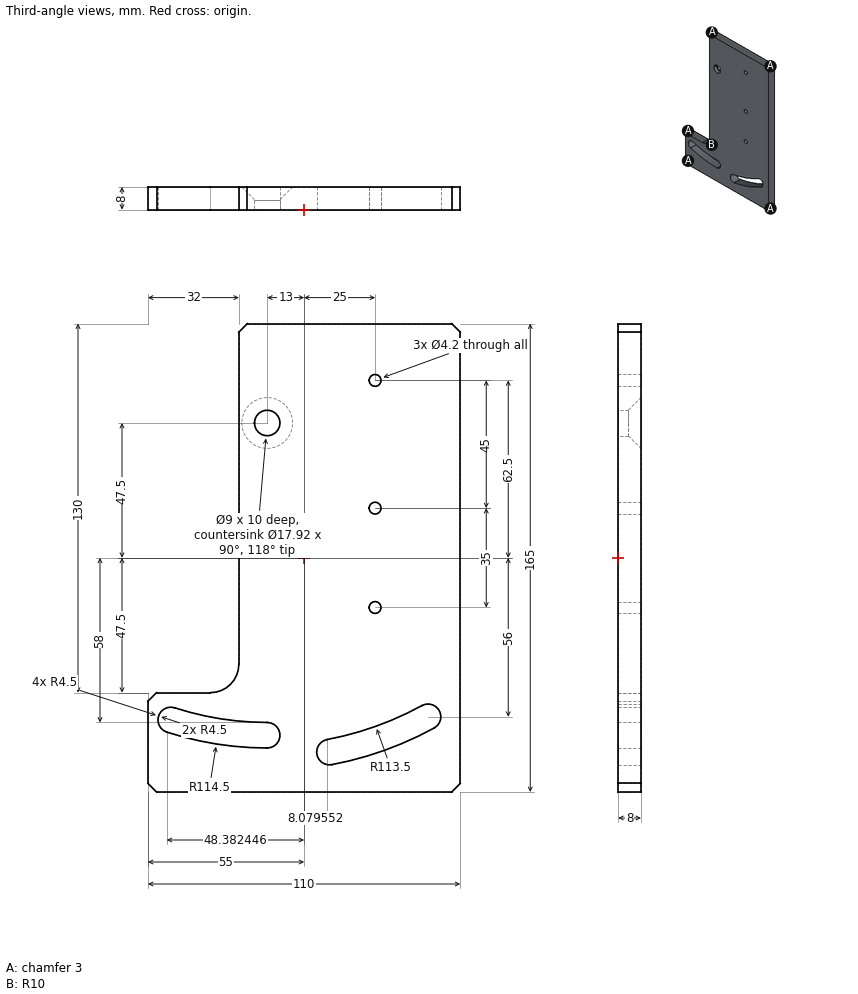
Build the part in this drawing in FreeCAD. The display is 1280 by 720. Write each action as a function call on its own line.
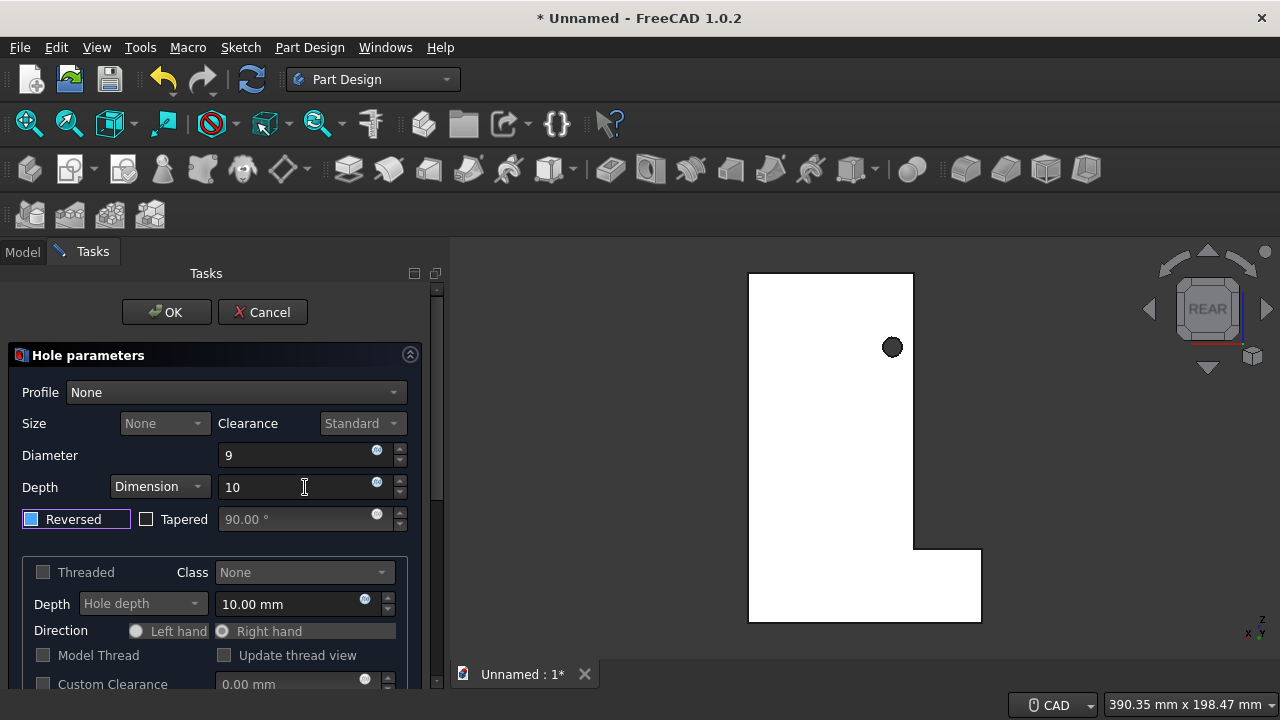
scroll(437, 486, down, 3)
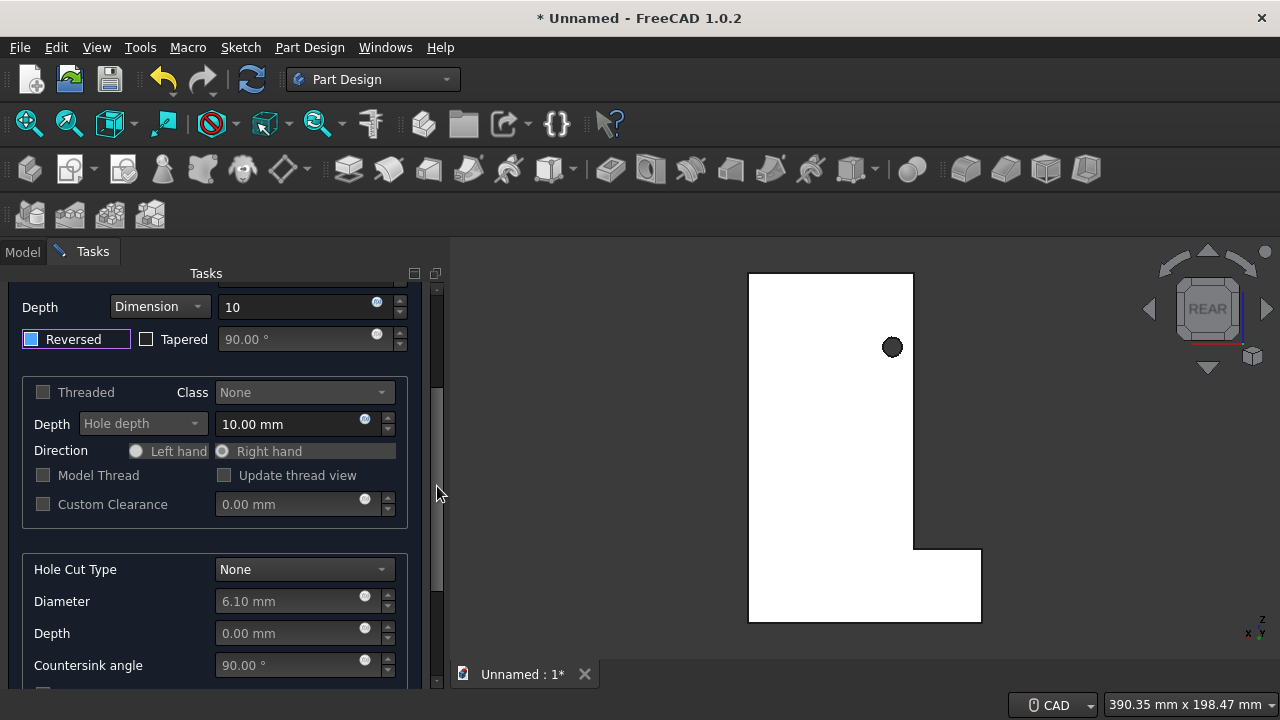
click(306, 570)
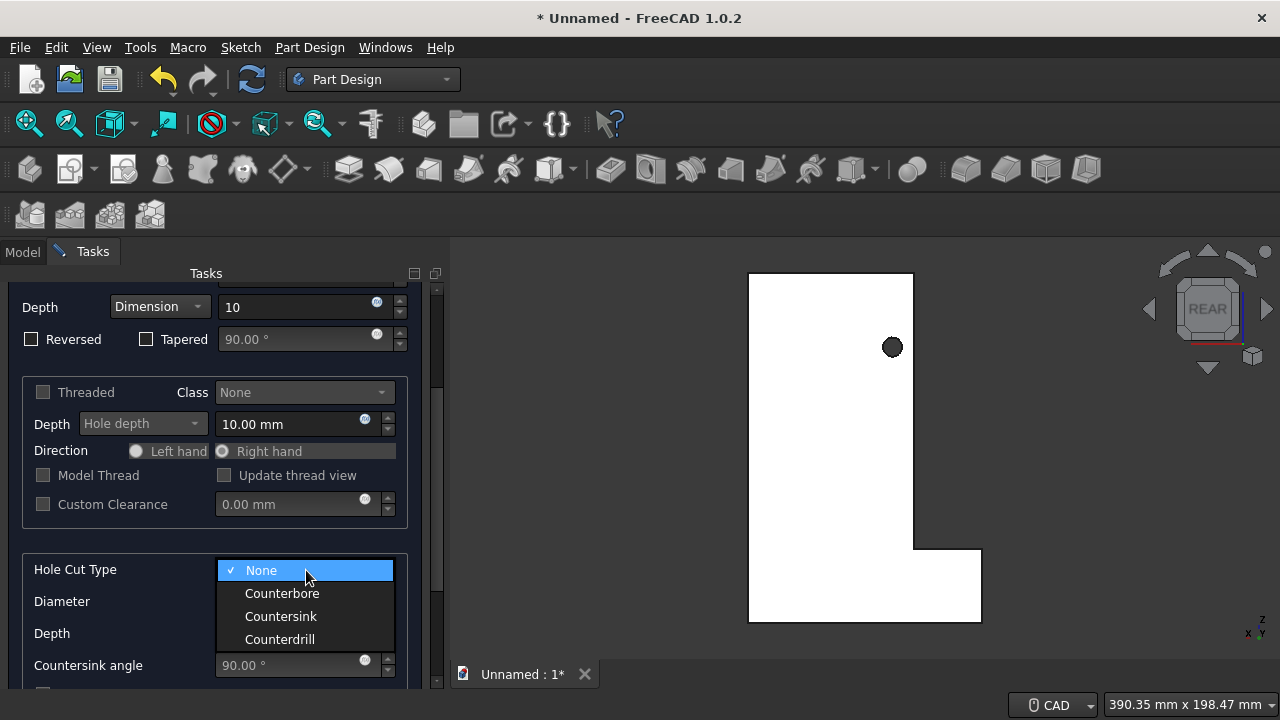
click(304, 616)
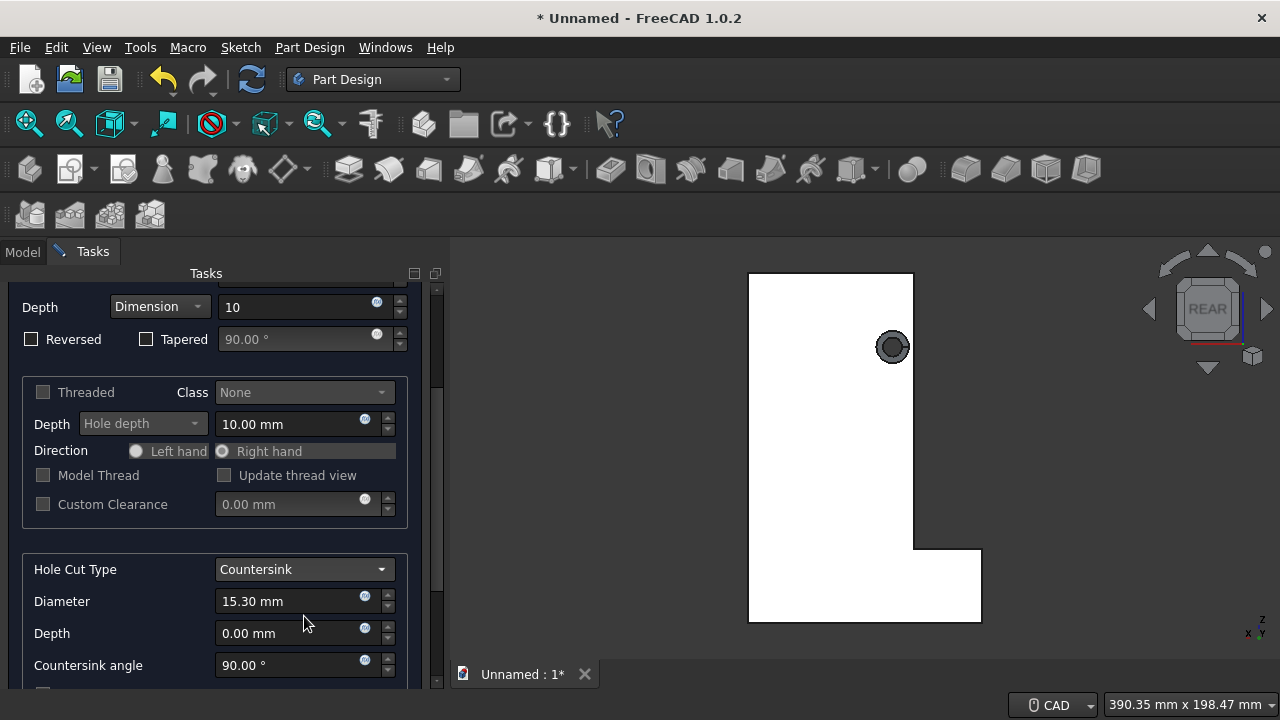
triple_click(298, 601)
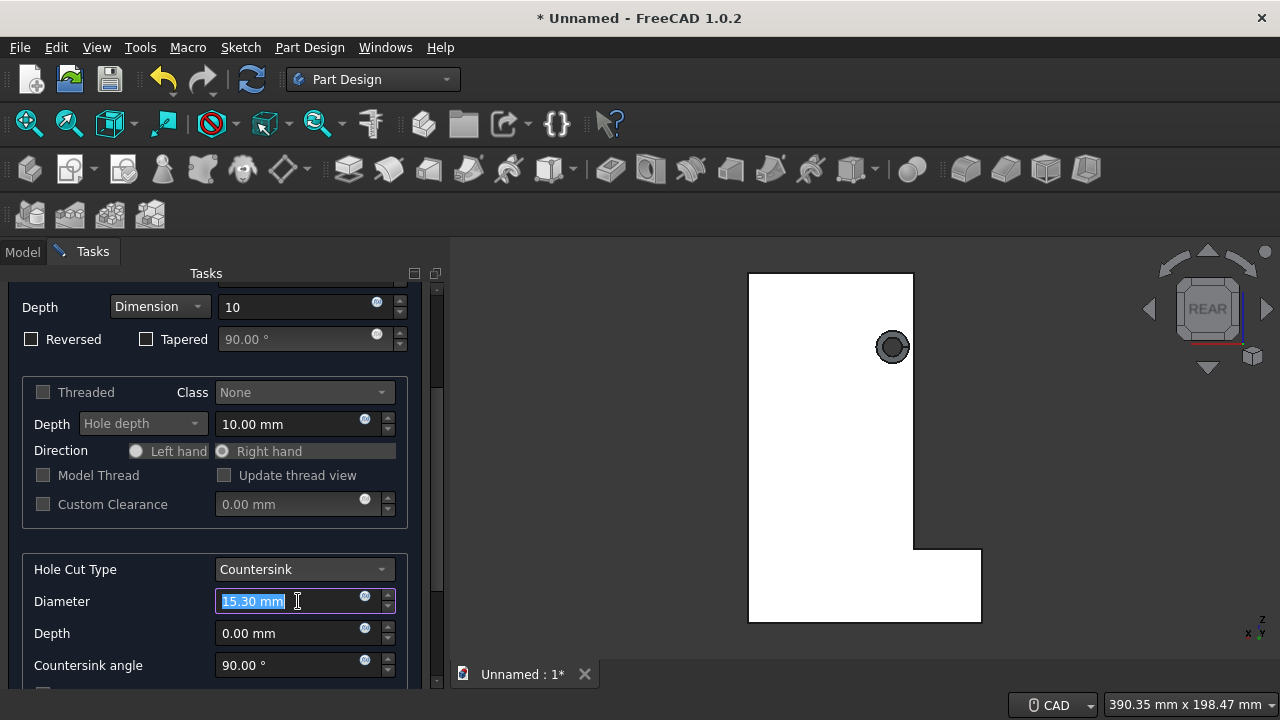
text(17.92)
key(Tab)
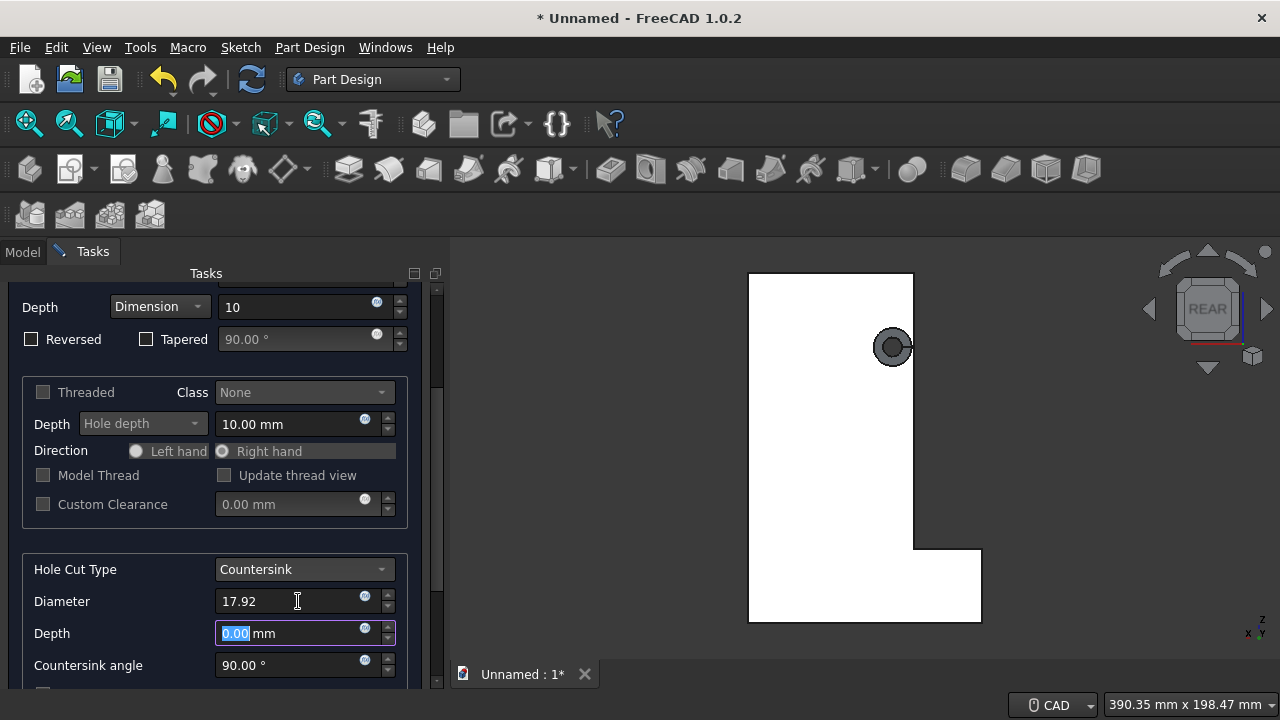
scroll(437, 486, up, 4)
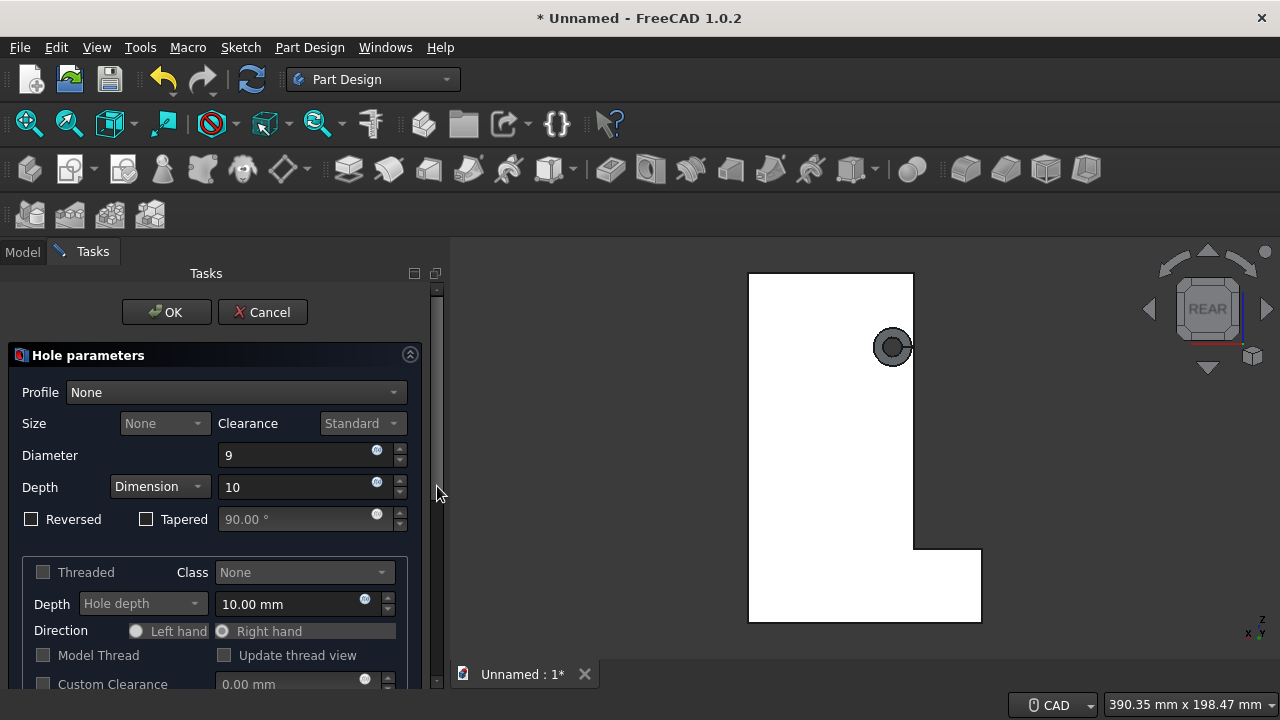
click(167, 312)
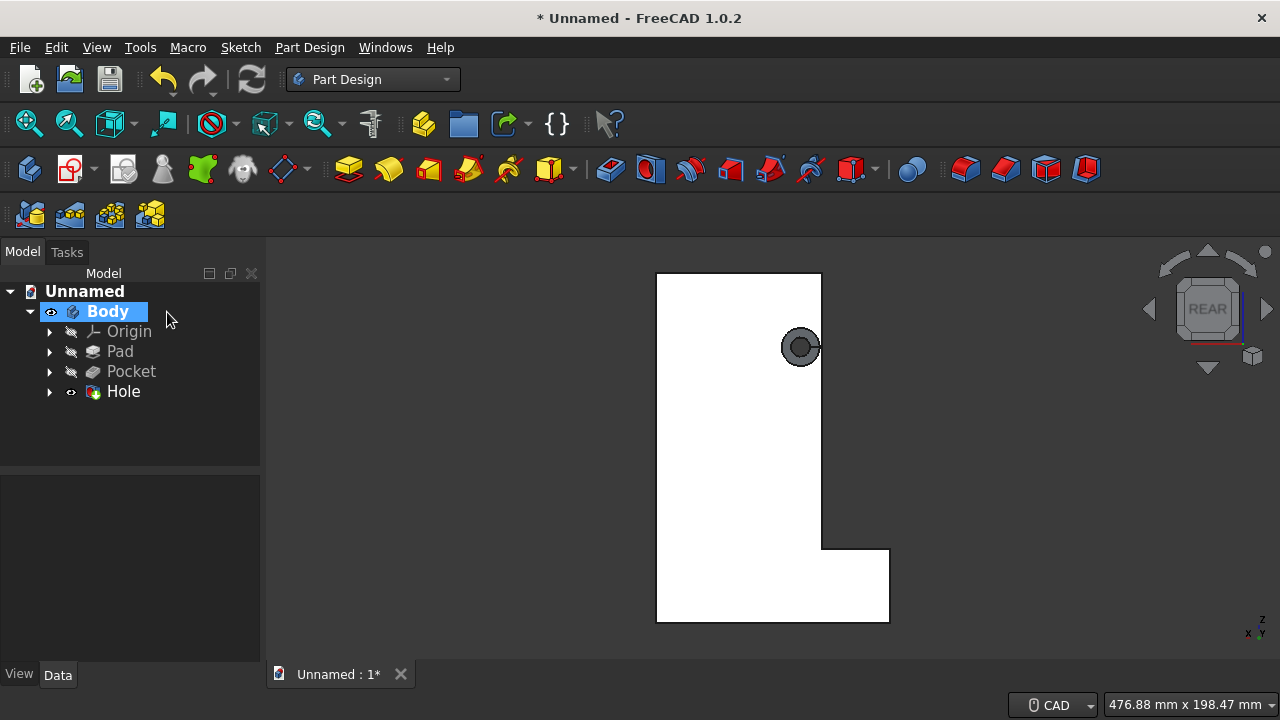
click(740, 447)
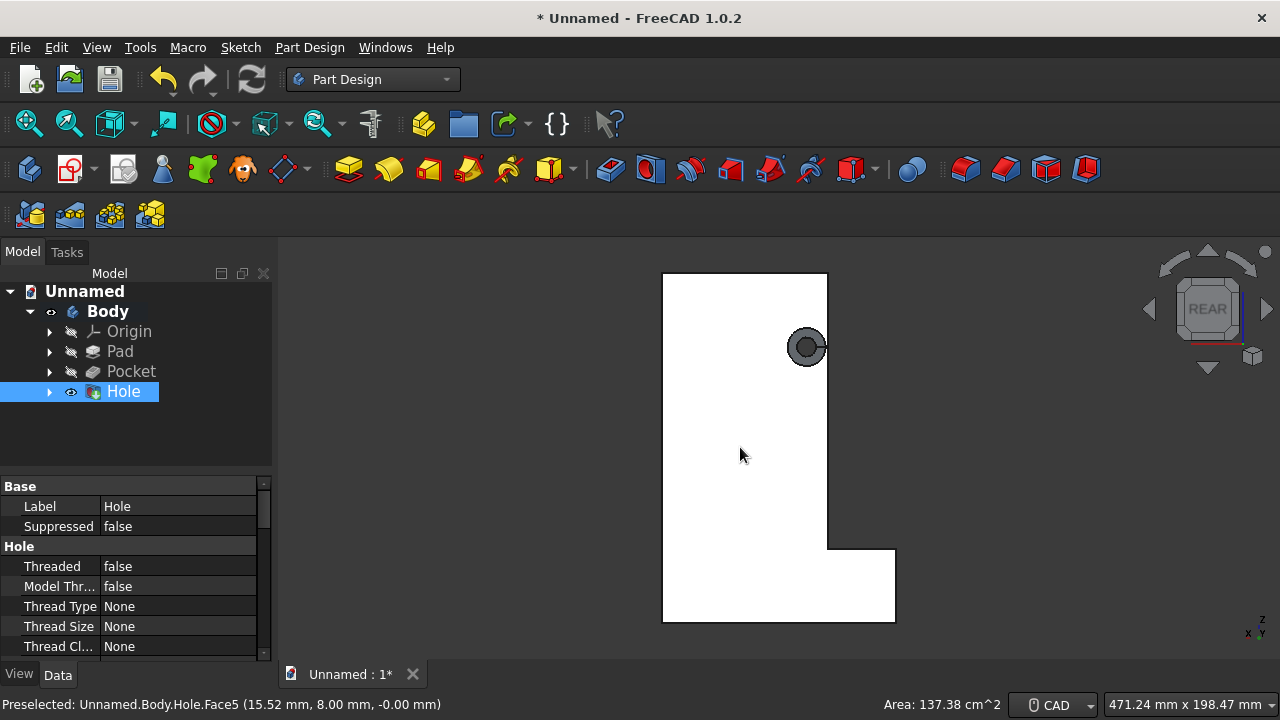
click(70, 170)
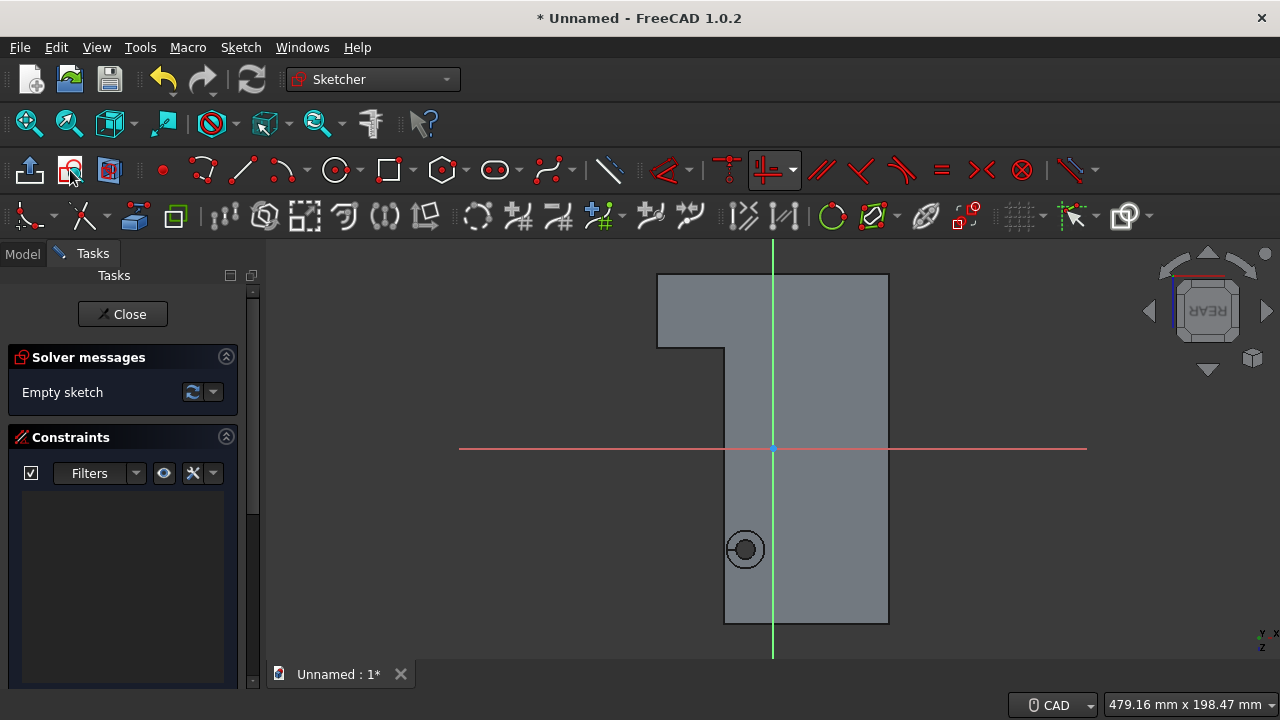
scroll(736, 292, up, 3)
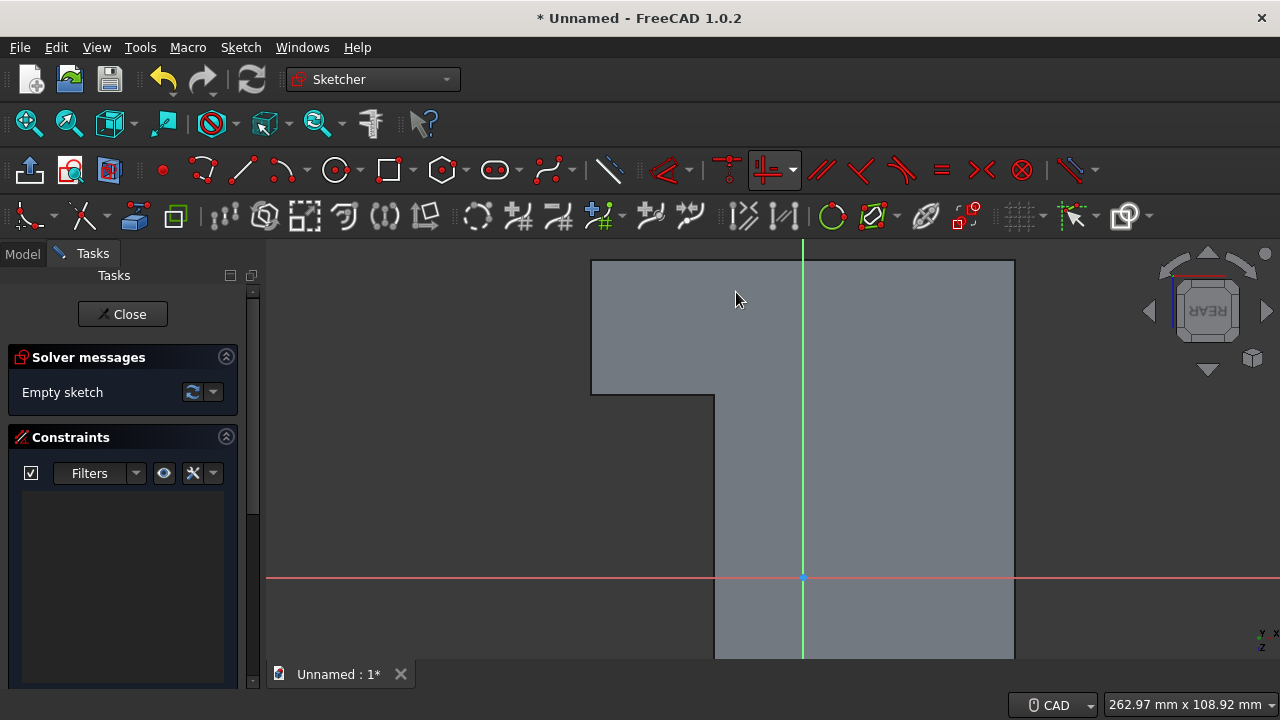
click(310, 170)